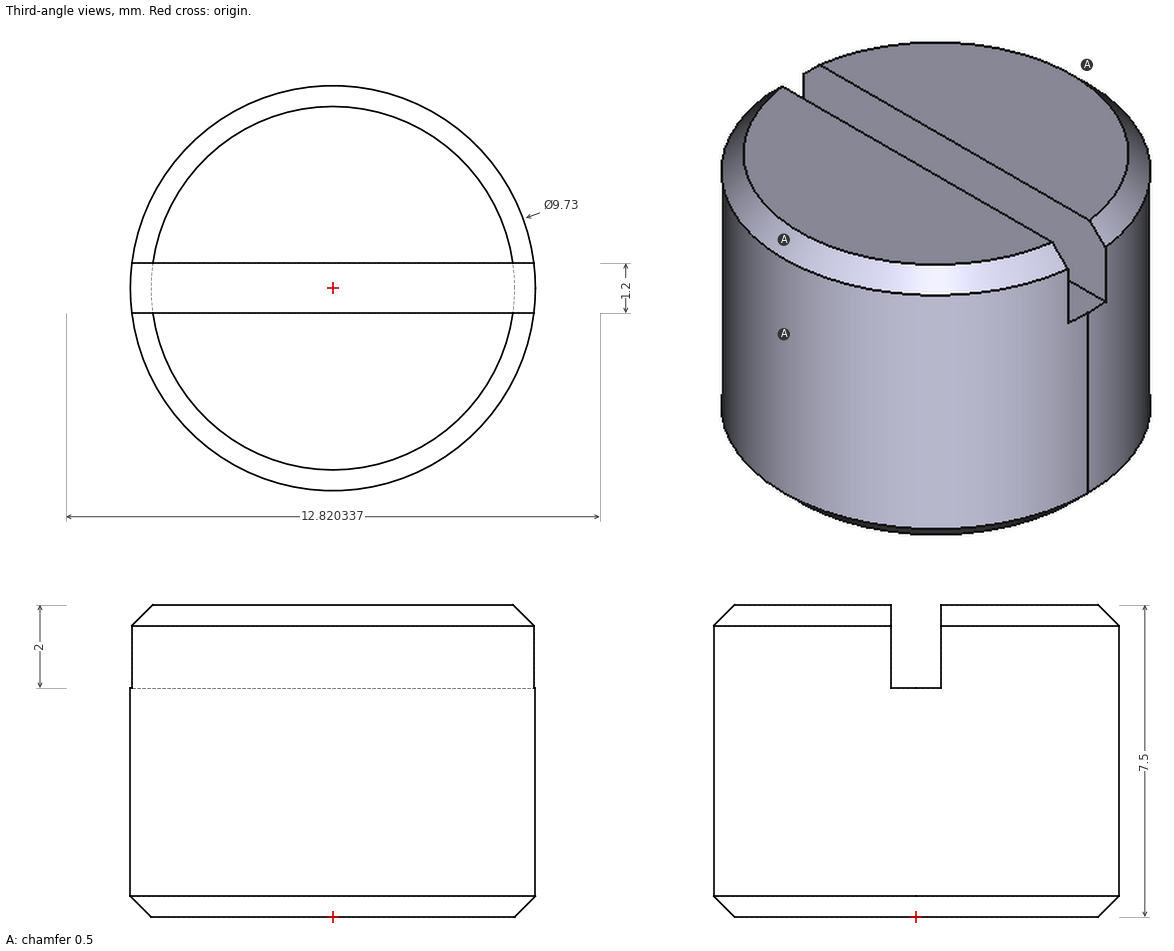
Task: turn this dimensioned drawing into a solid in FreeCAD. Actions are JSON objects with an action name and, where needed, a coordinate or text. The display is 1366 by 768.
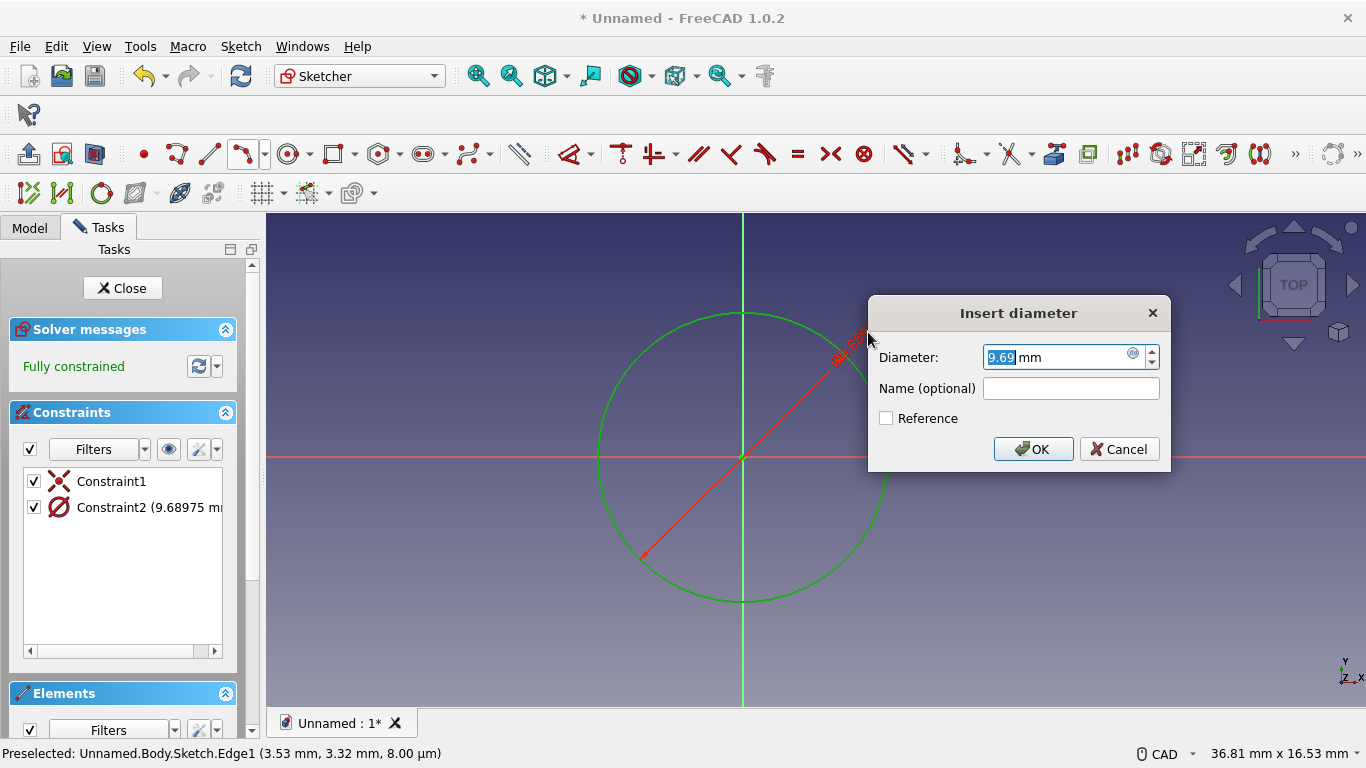
{"action": "type", "text": "9.73"}
{"action": "key", "text": "Return"}
{"action": "key", "text": "Escape"}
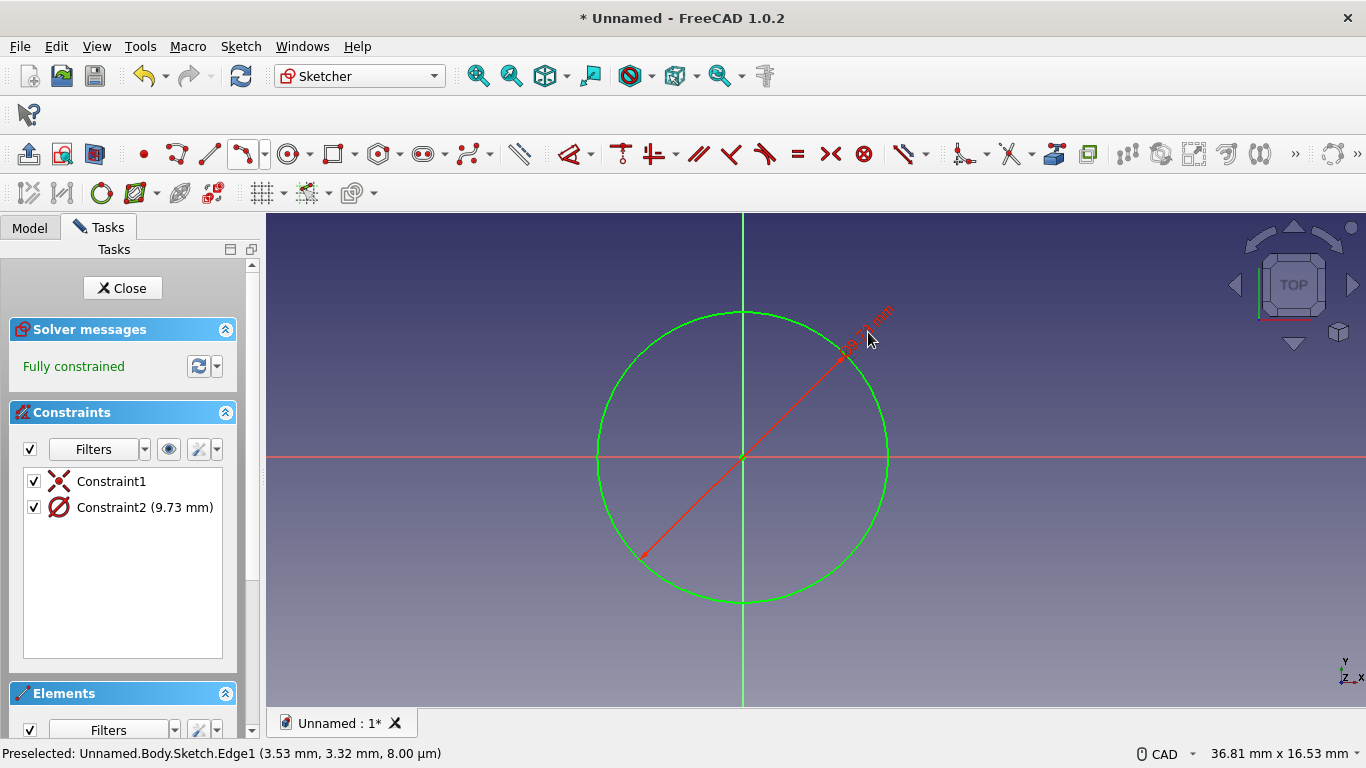
{"action": "left_click", "coordinate": [123, 288]}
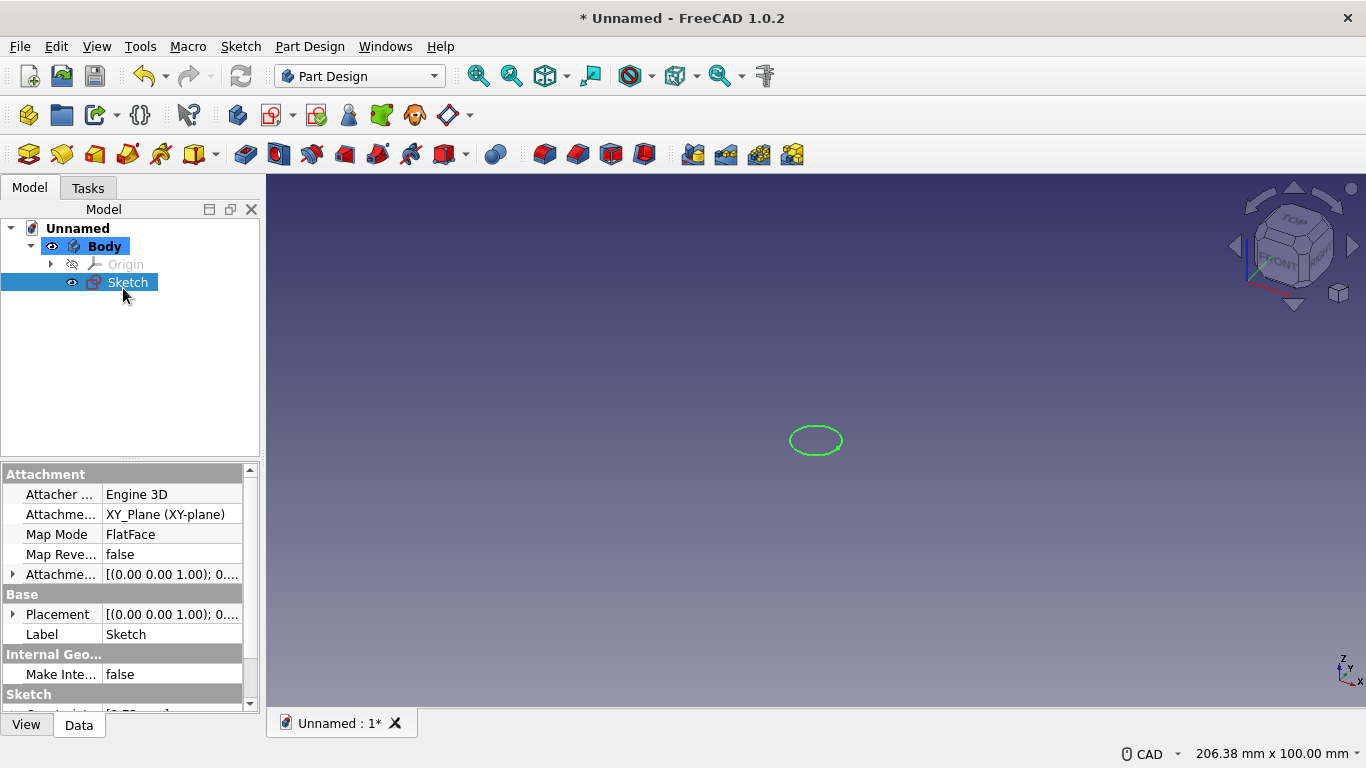
{"action": "left_click", "coordinate": [29, 154]}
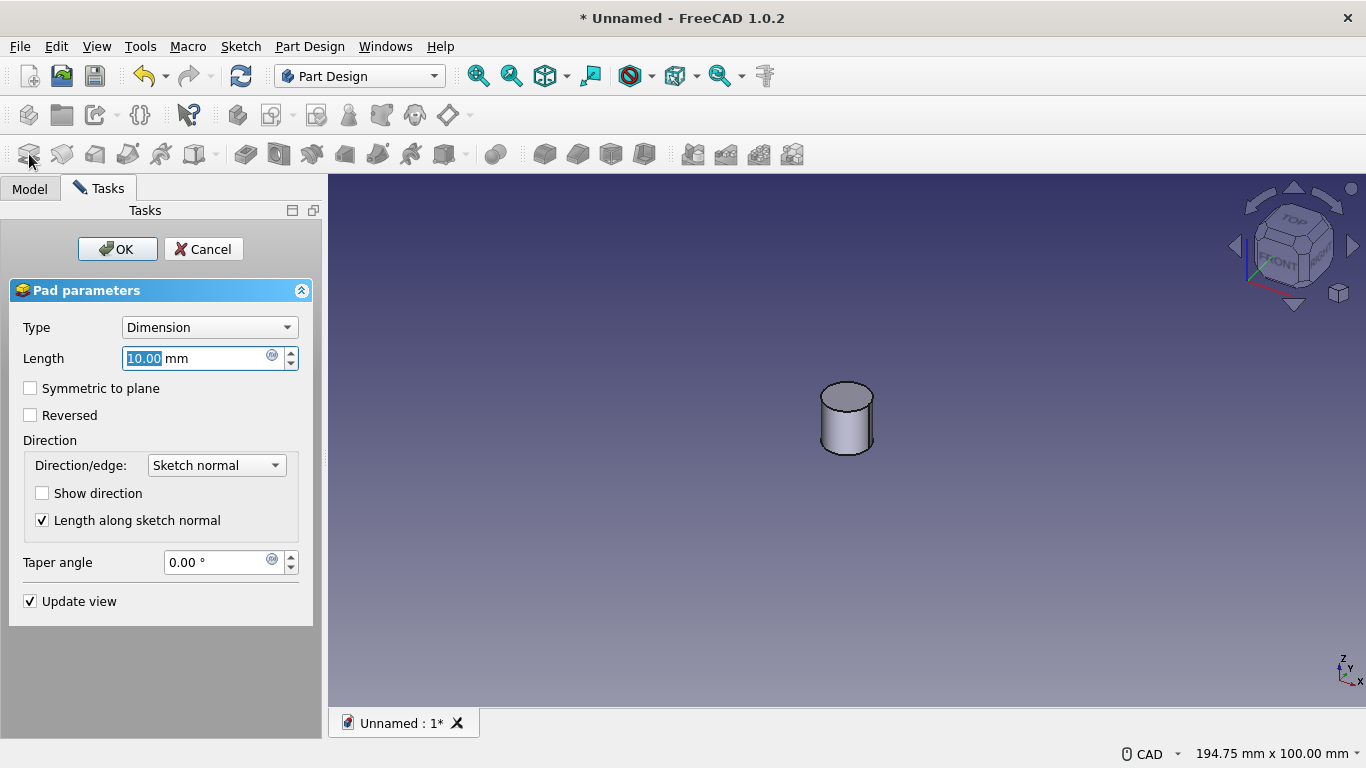
{"action": "type", "text": "7.5"}
{"action": "key", "text": "Tab"}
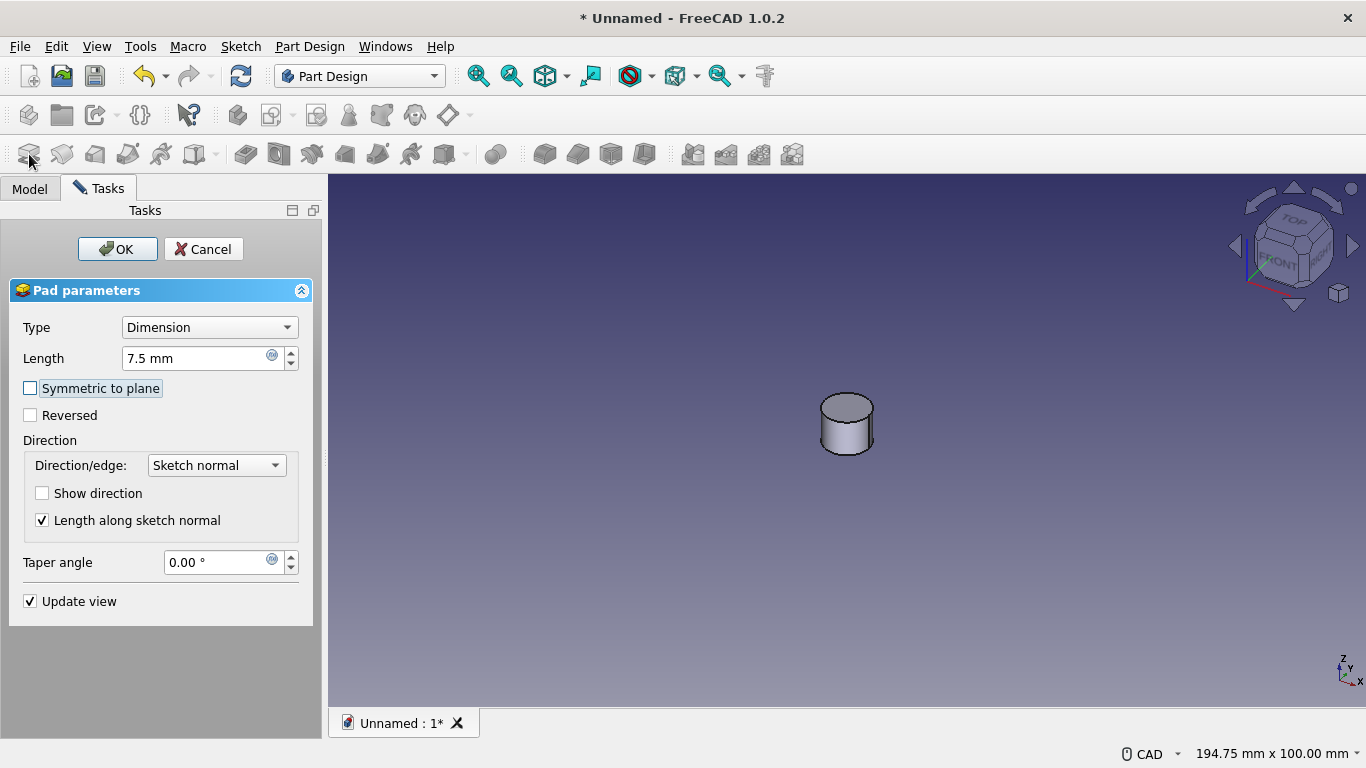
{"action": "left_click", "coordinate": [118, 249]}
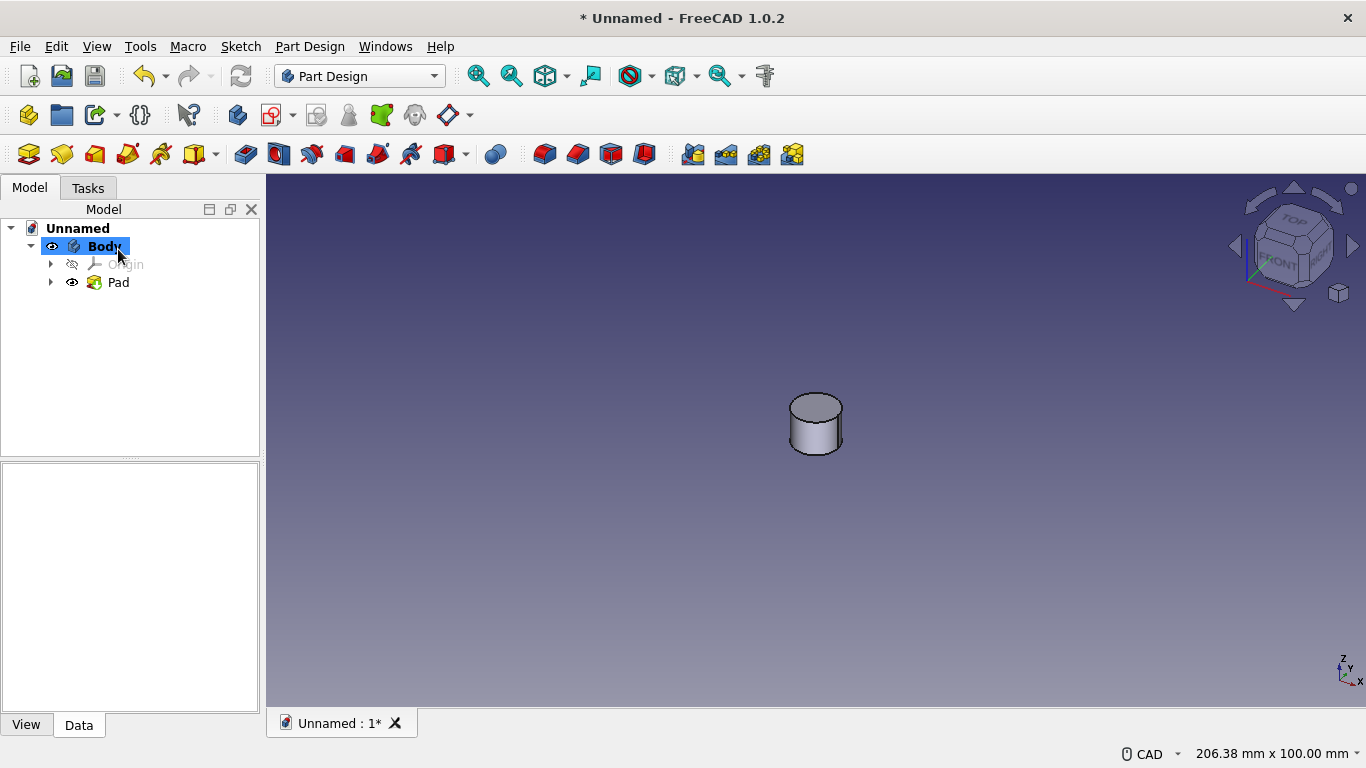
{"action": "left_click", "coordinate": [479, 76]}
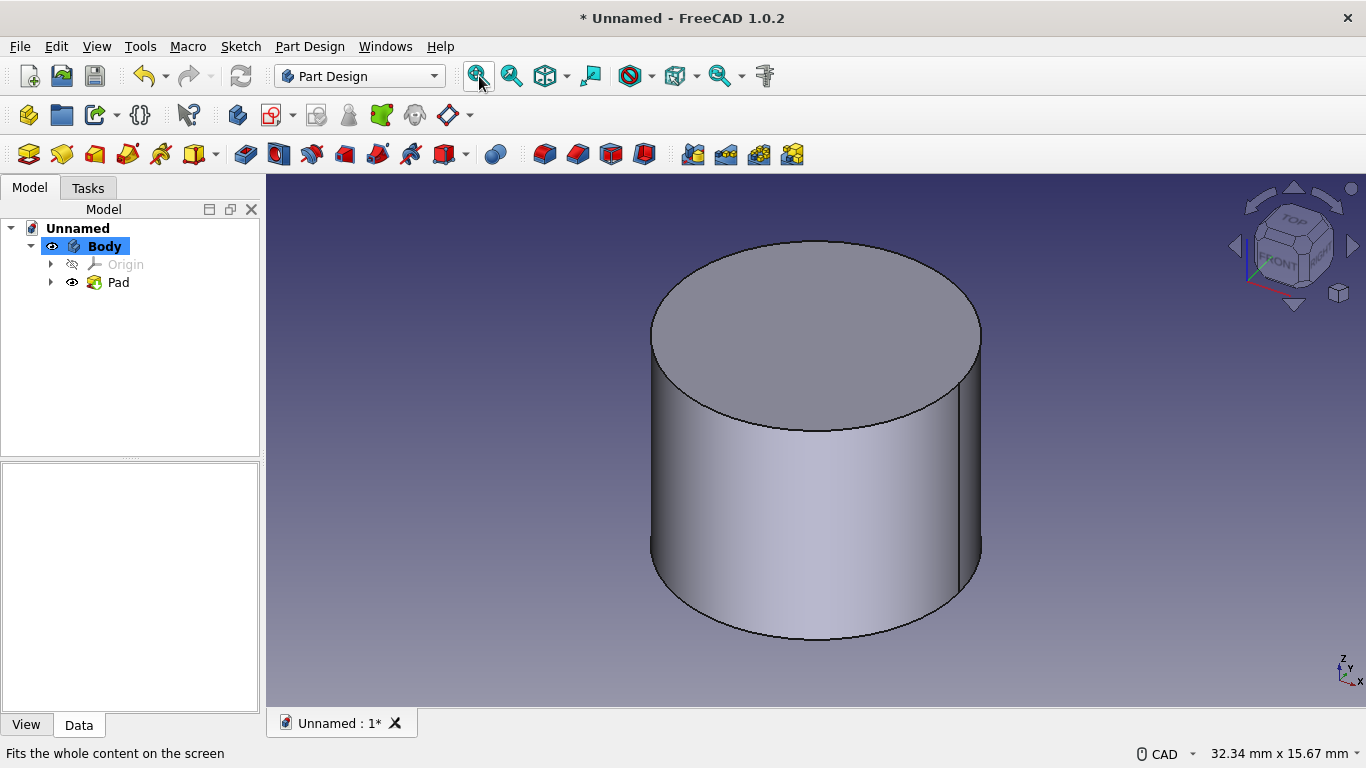
{"action": "left_click", "coordinate": [816, 335]}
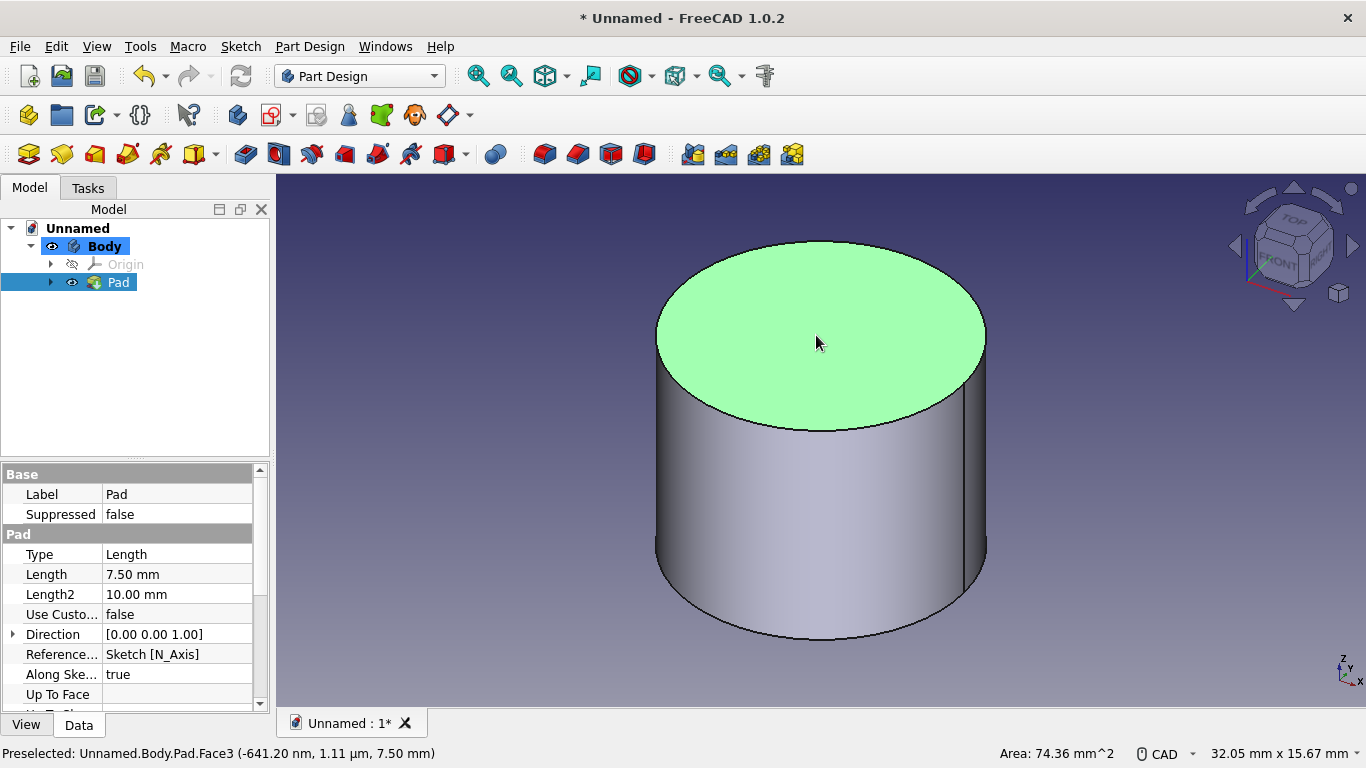
{"action": "left_click", "coordinate": [270, 116]}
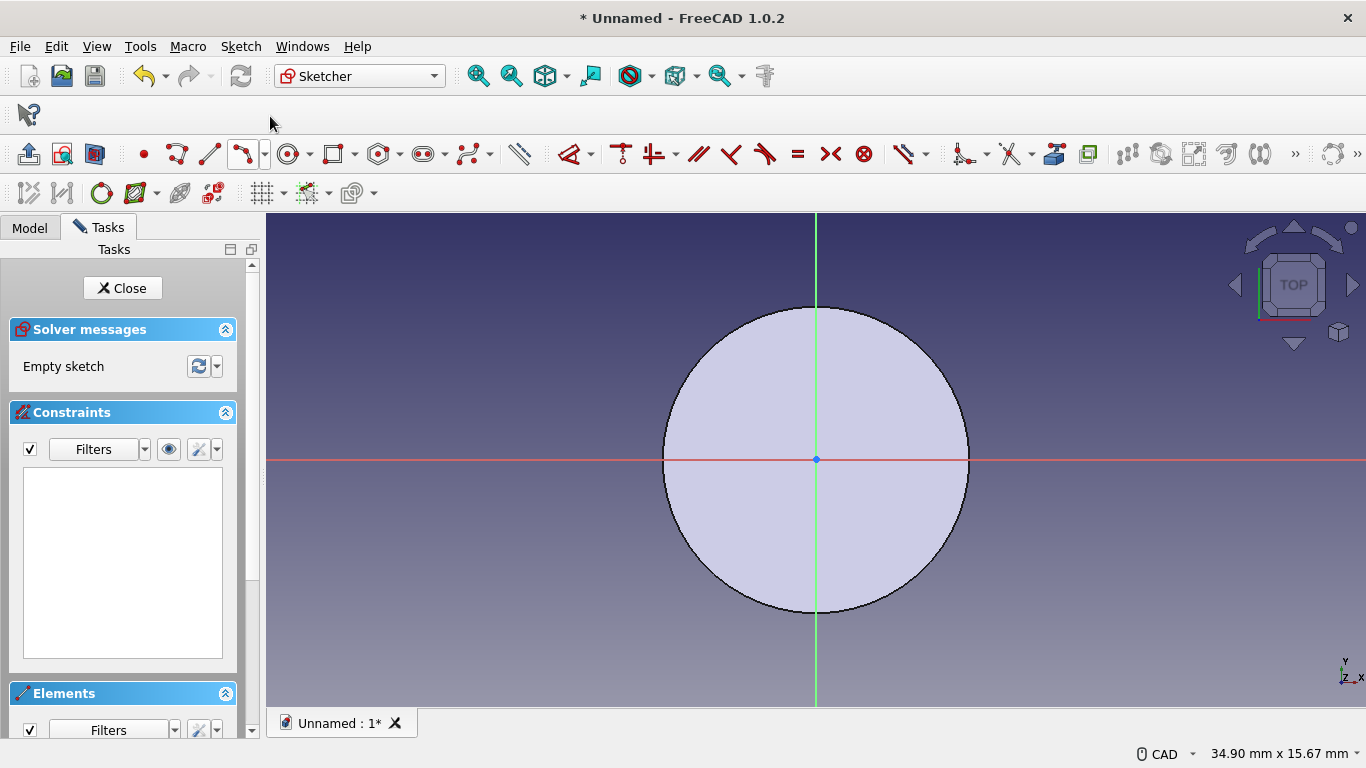
{"action": "scroll", "coordinate": [955, 460], "scroll_direction": "up", "scroll_amount": 2}